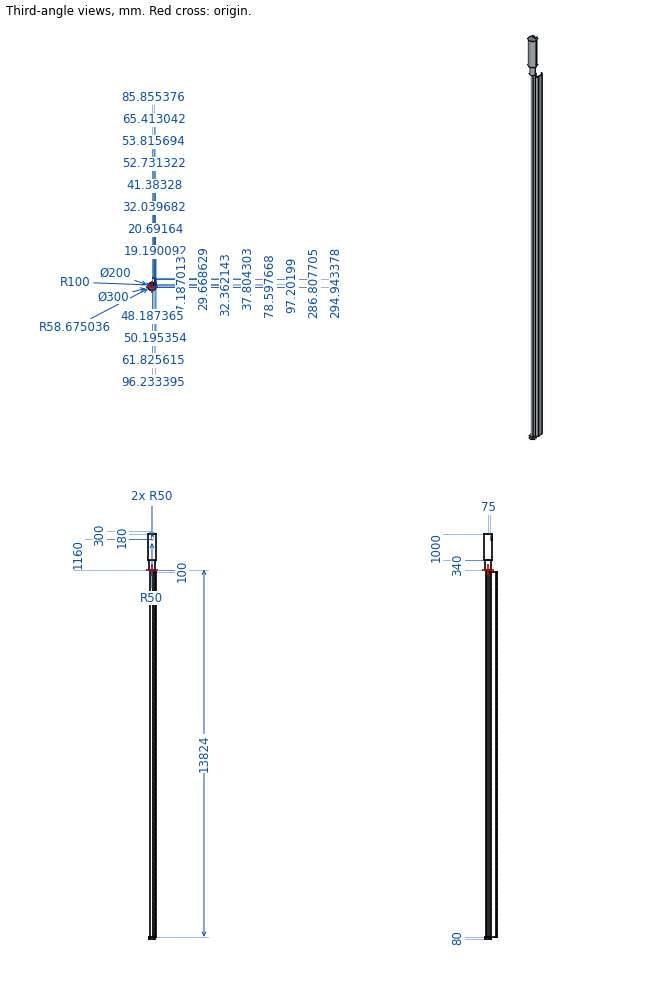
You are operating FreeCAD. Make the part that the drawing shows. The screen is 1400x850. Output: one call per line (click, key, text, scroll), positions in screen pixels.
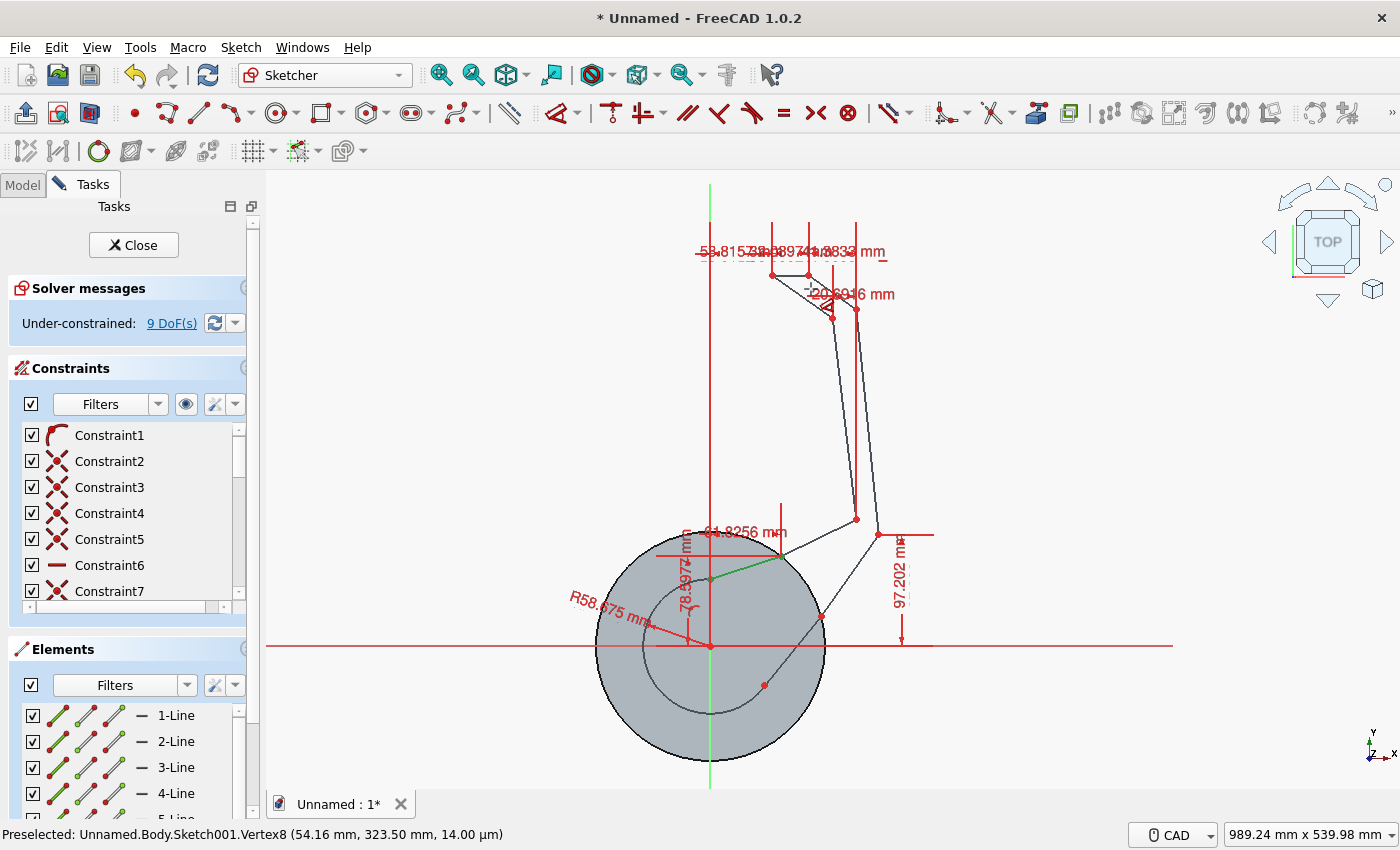
click(821, 616)
click(740, 680)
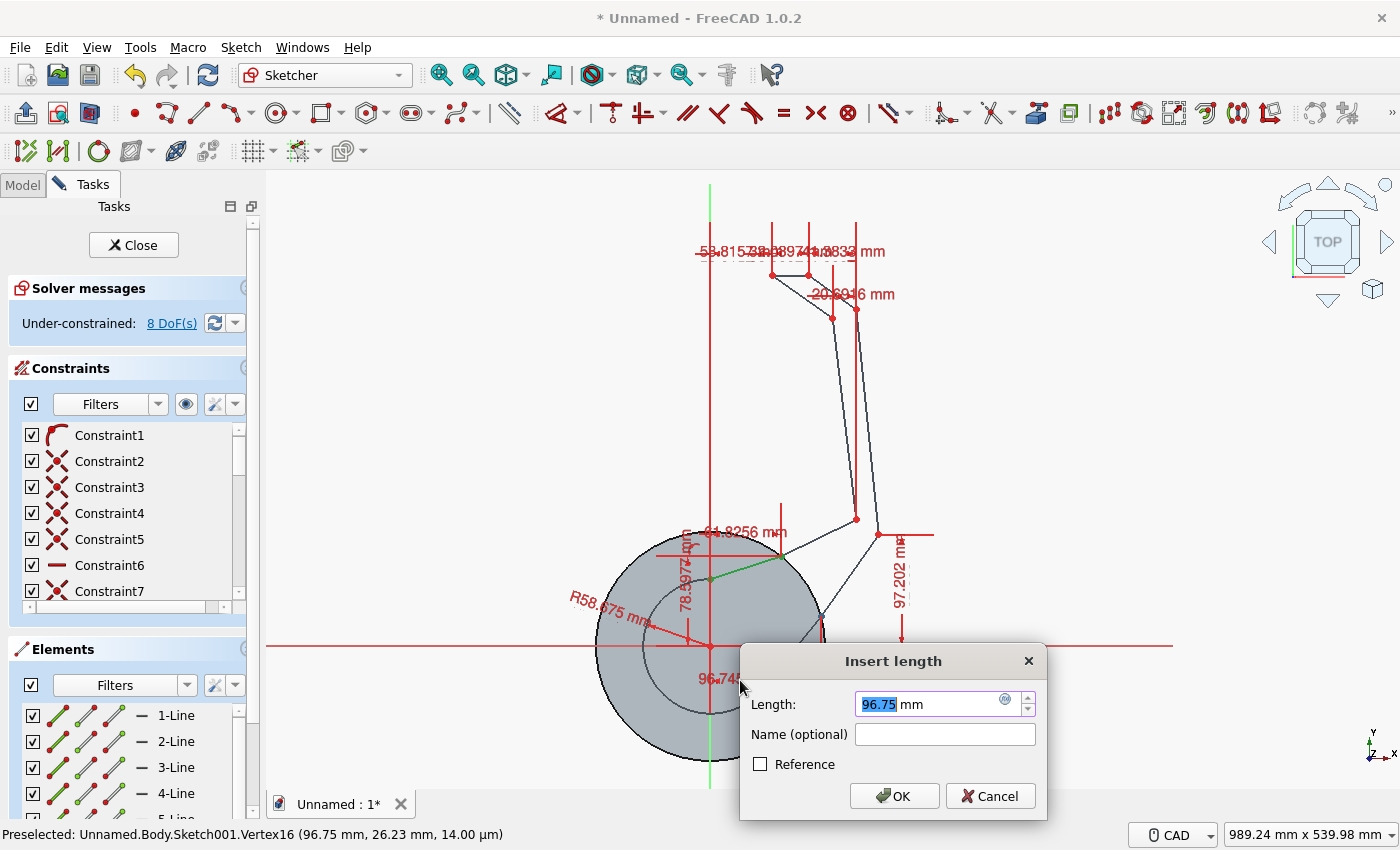
text(96.233395)
key(Return)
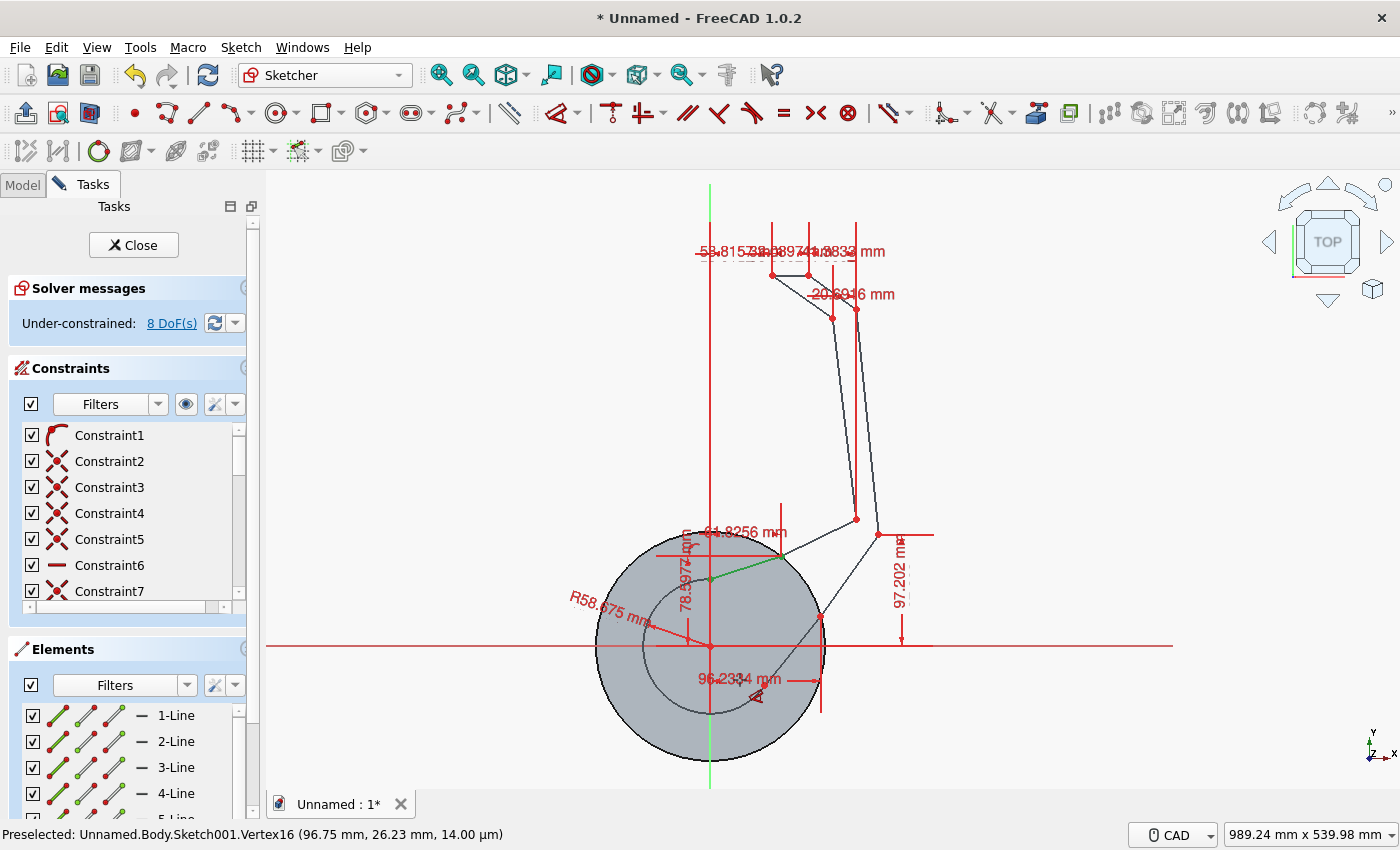
scroll(821, 616, up, 2)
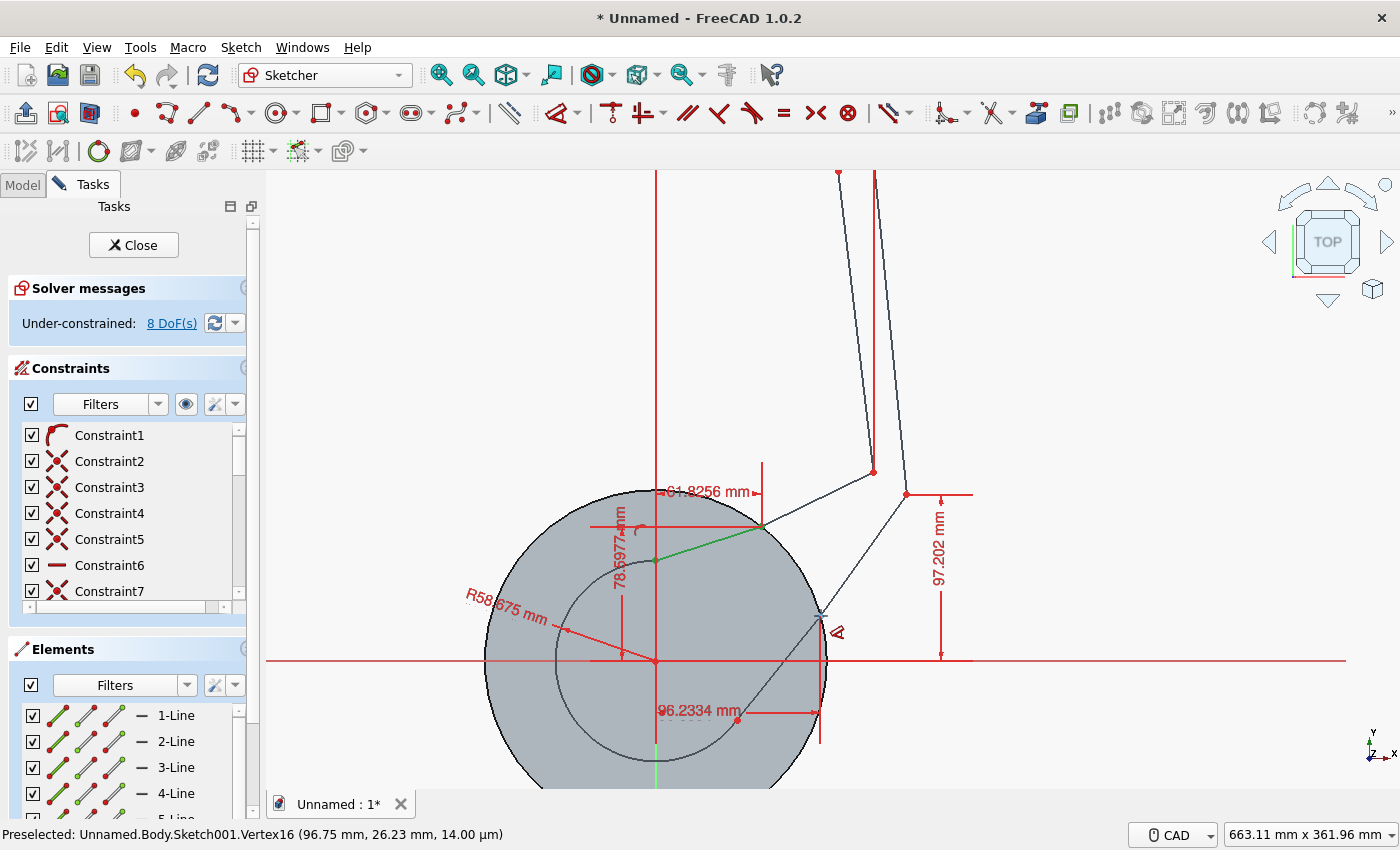
click(820, 616)
click(854, 639)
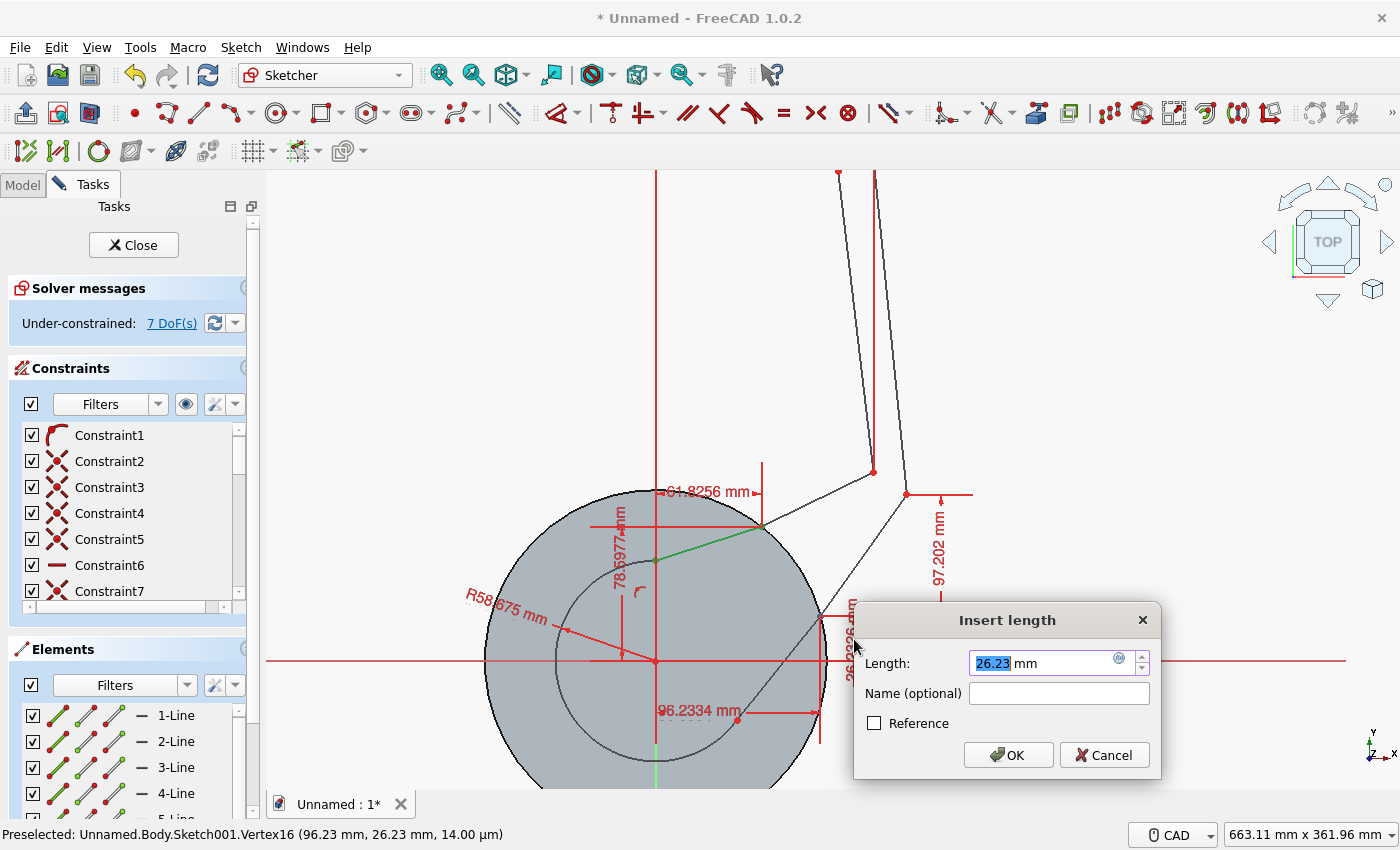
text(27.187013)
key(Return)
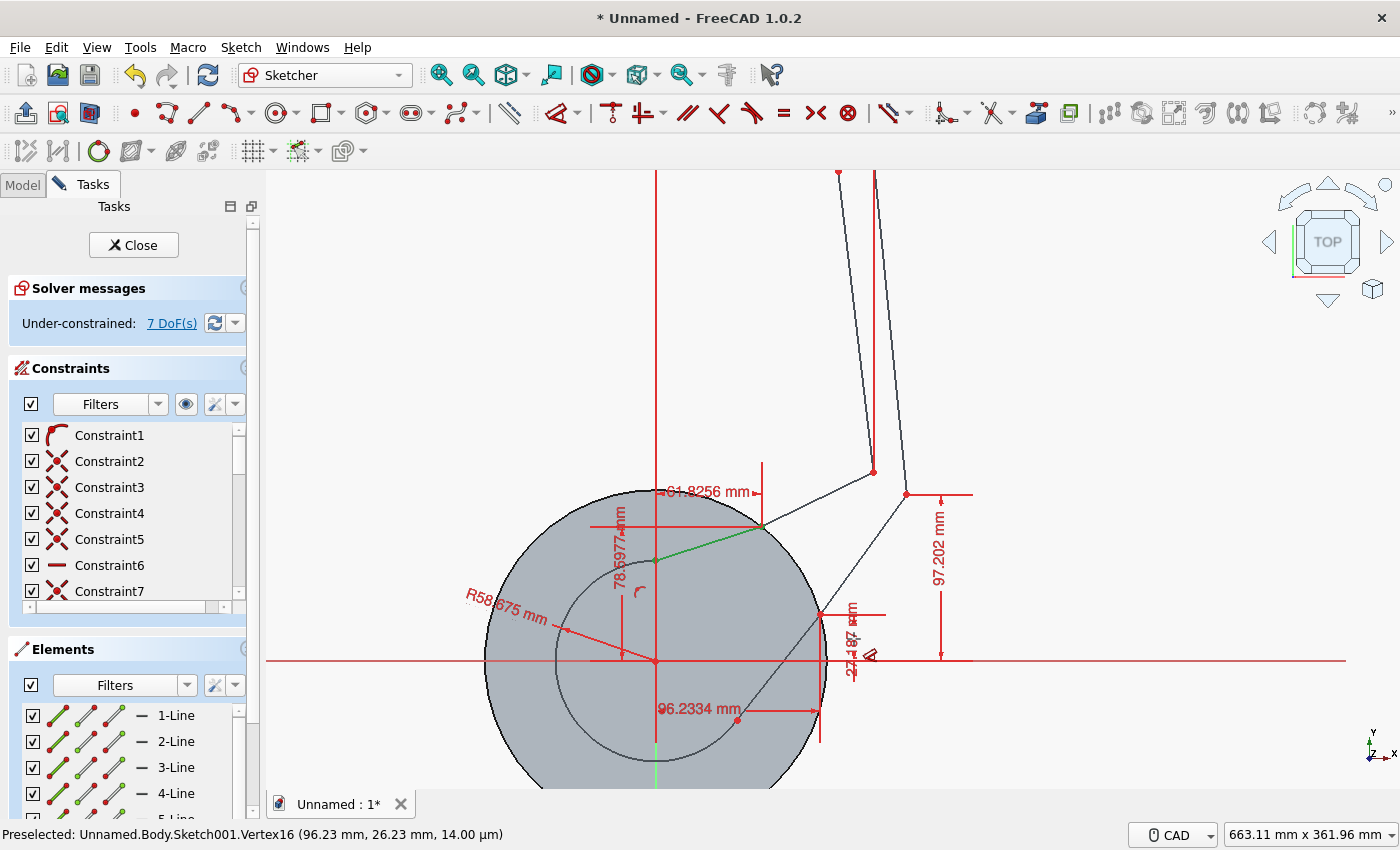
click(737, 720)
click(725, 754)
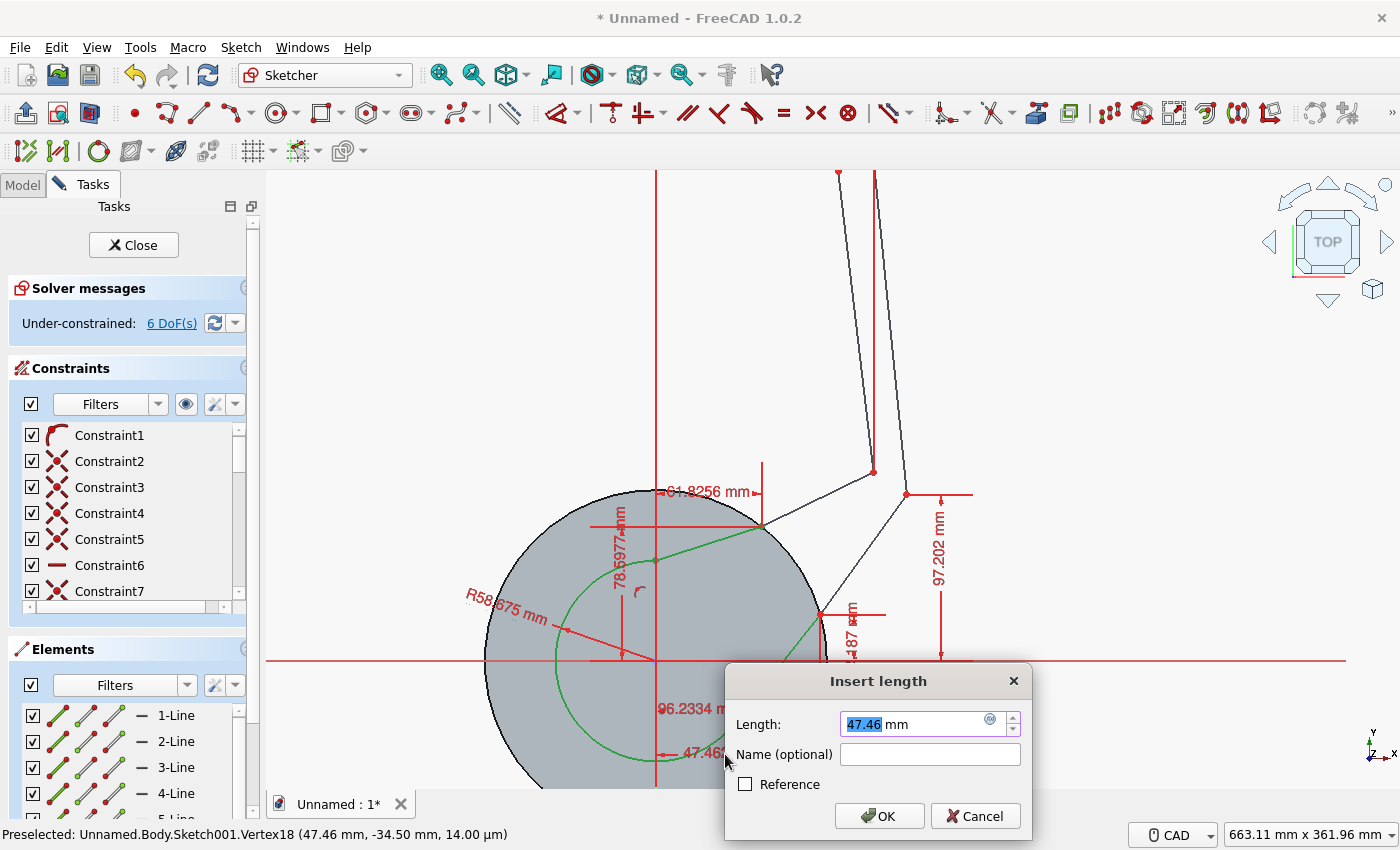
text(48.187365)
key(Return)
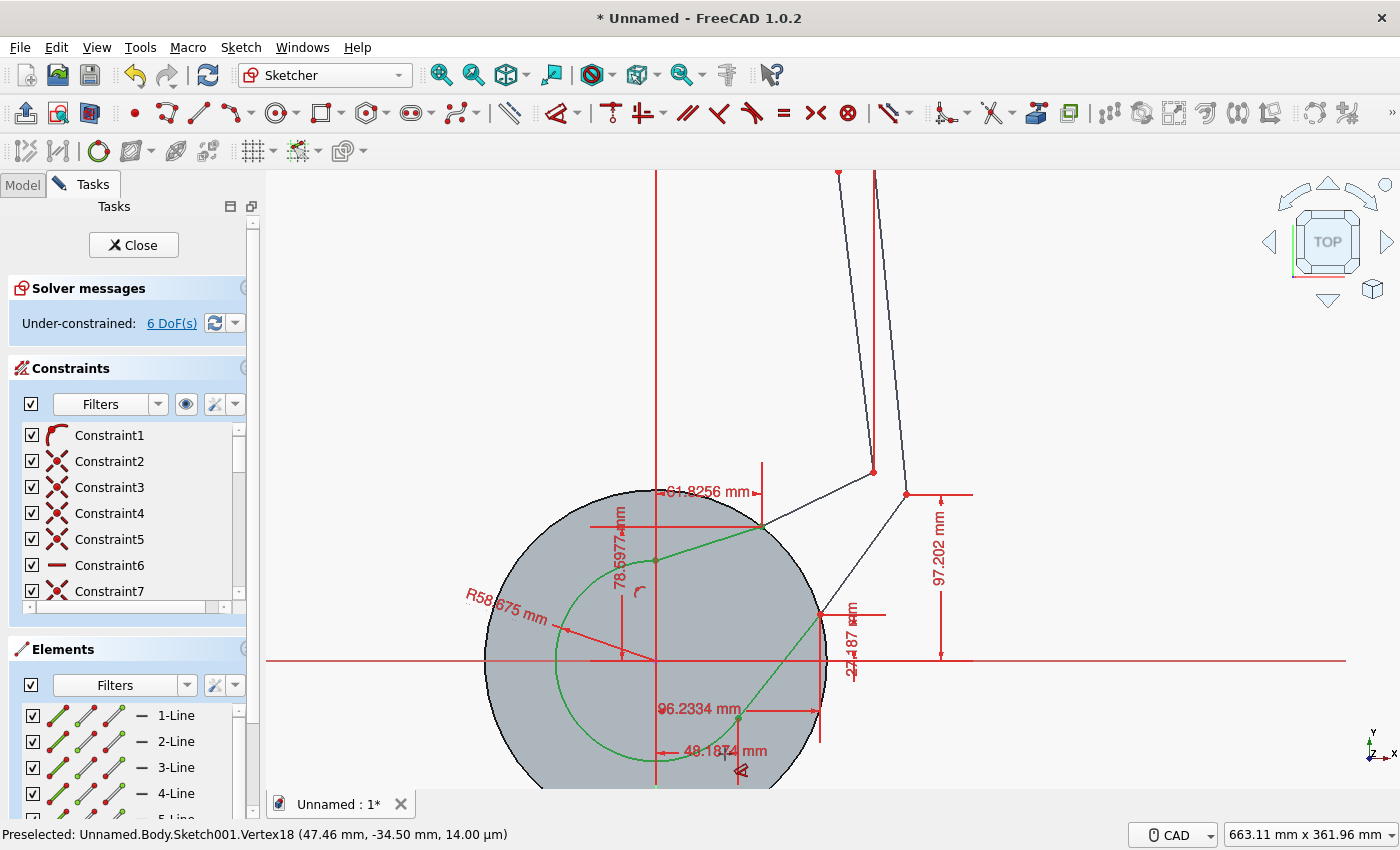
click(795, 510)
click(818, 561)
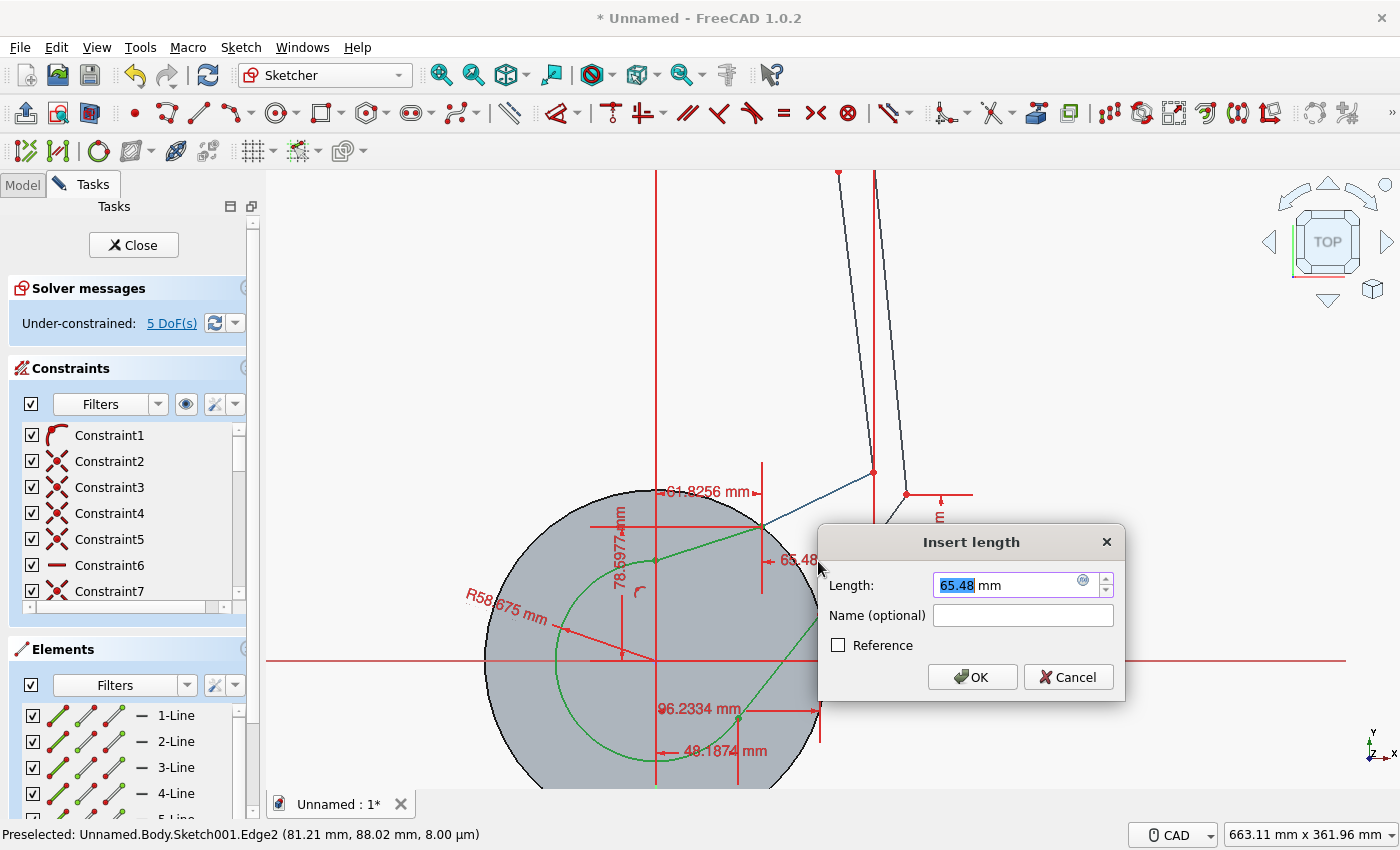
text(65.413042)
key(Return)